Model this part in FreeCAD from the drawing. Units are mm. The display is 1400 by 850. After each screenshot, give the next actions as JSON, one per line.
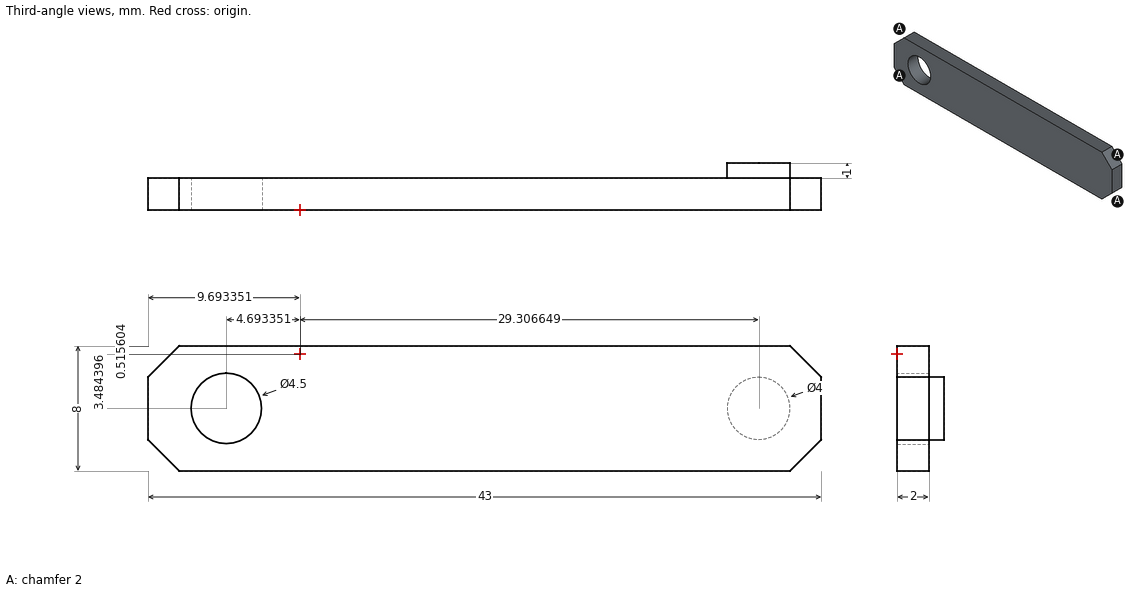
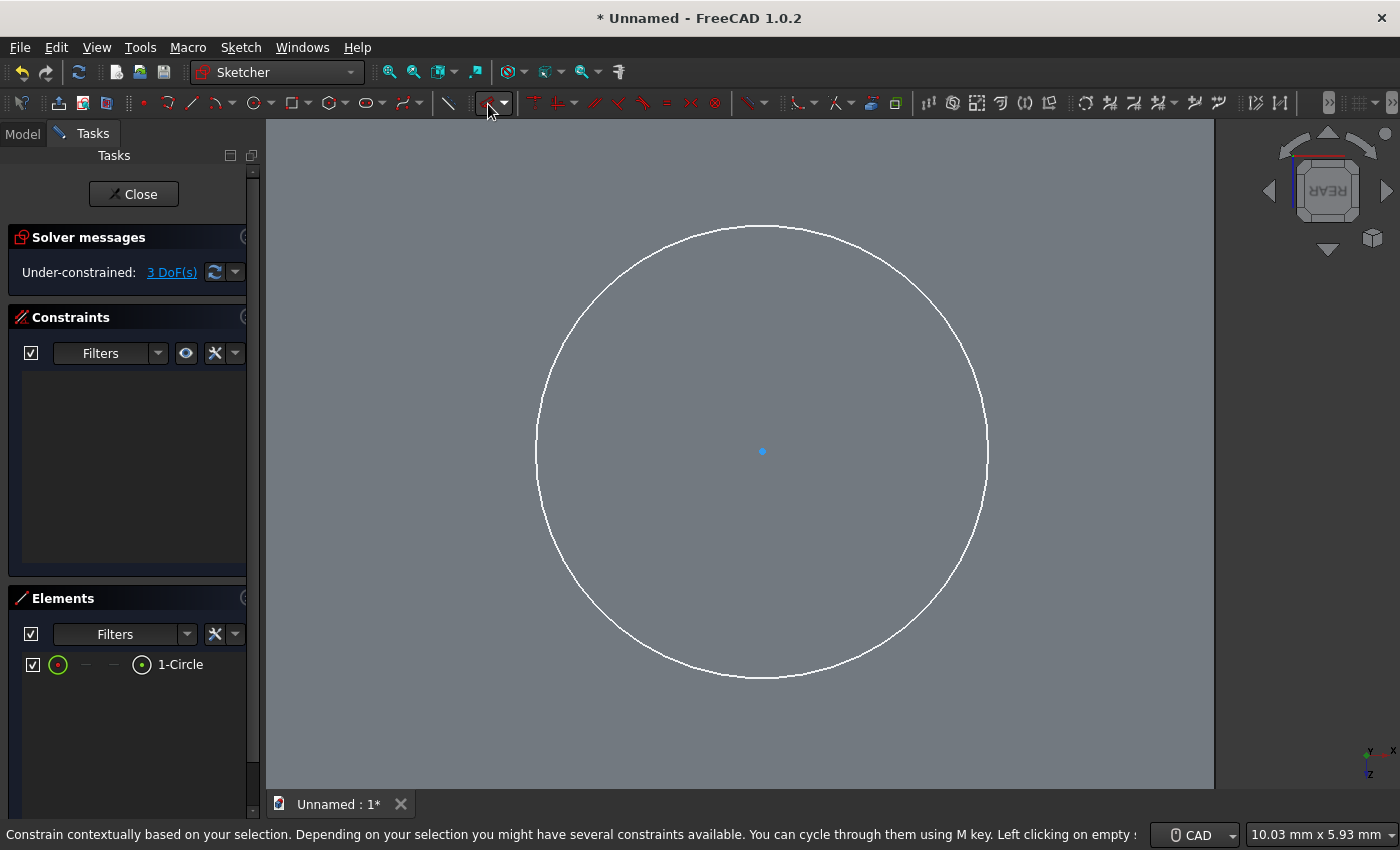
{"action": "left_click", "coordinate": [922, 292]}
{"action": "left_click", "coordinate": [945, 269]}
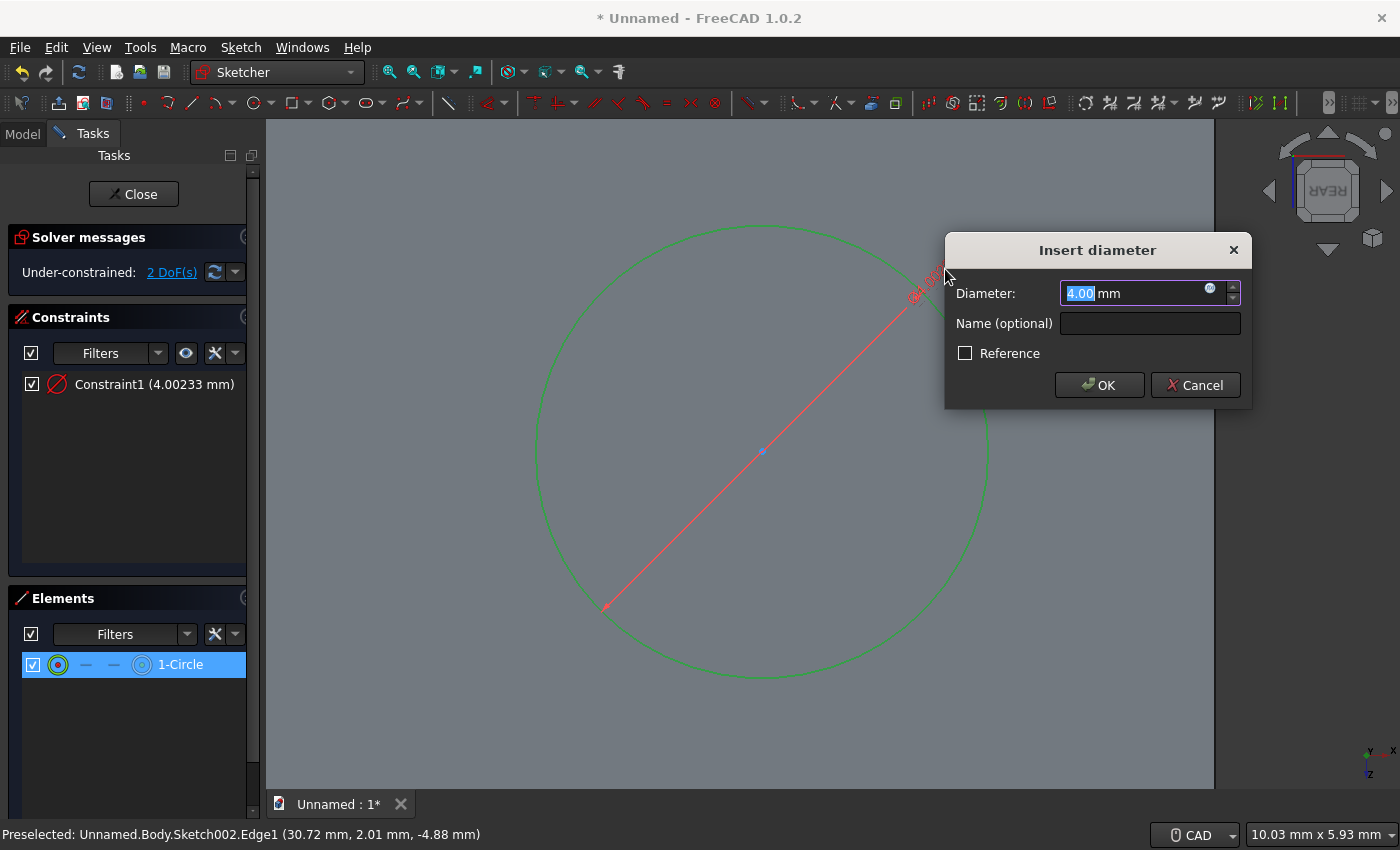
{"action": "type", "text": "4"}
{"action": "key", "text": "Return"}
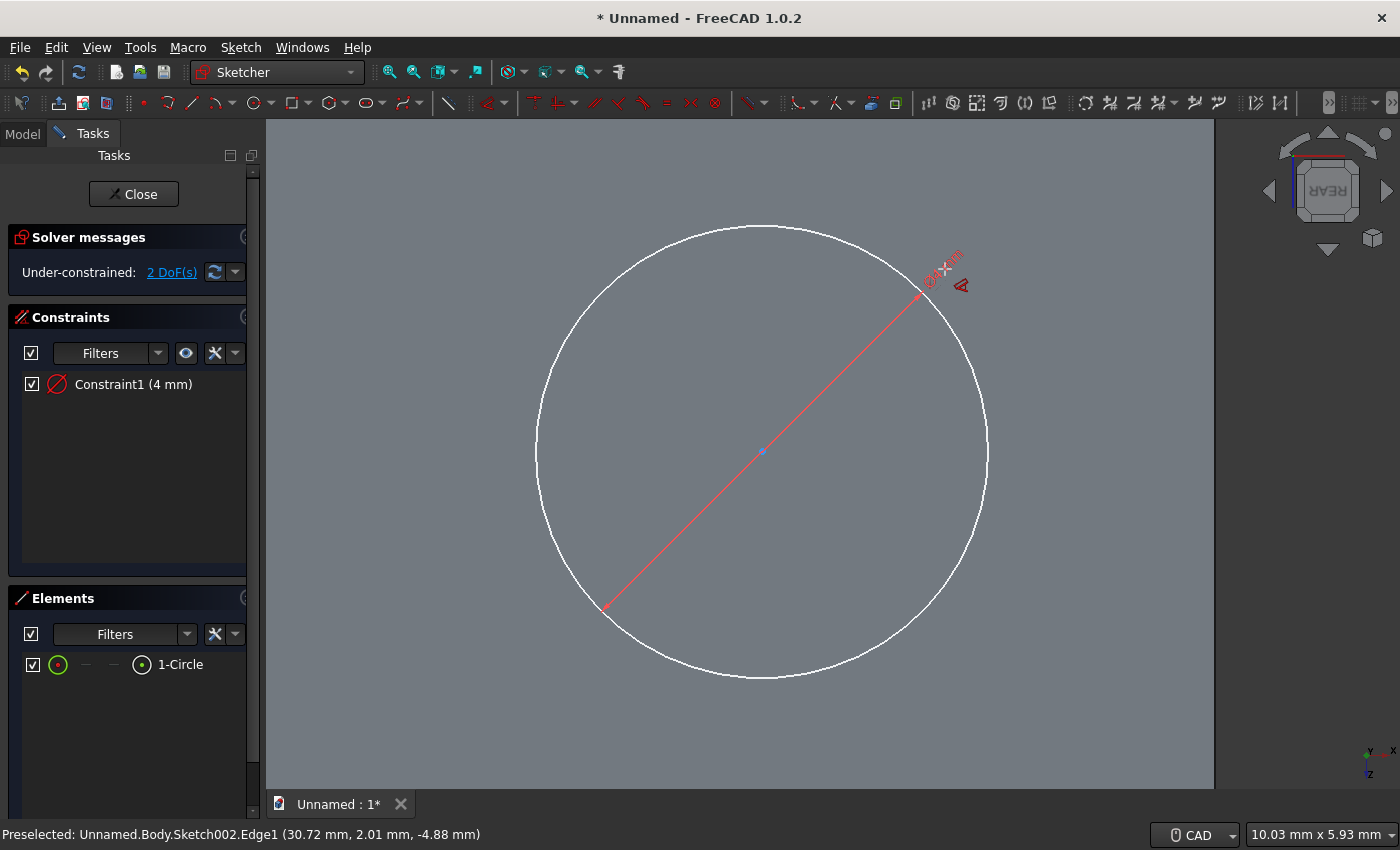
{"action": "left_click", "coordinate": [762, 452]}
{"action": "left_click", "coordinate": [796, 606]}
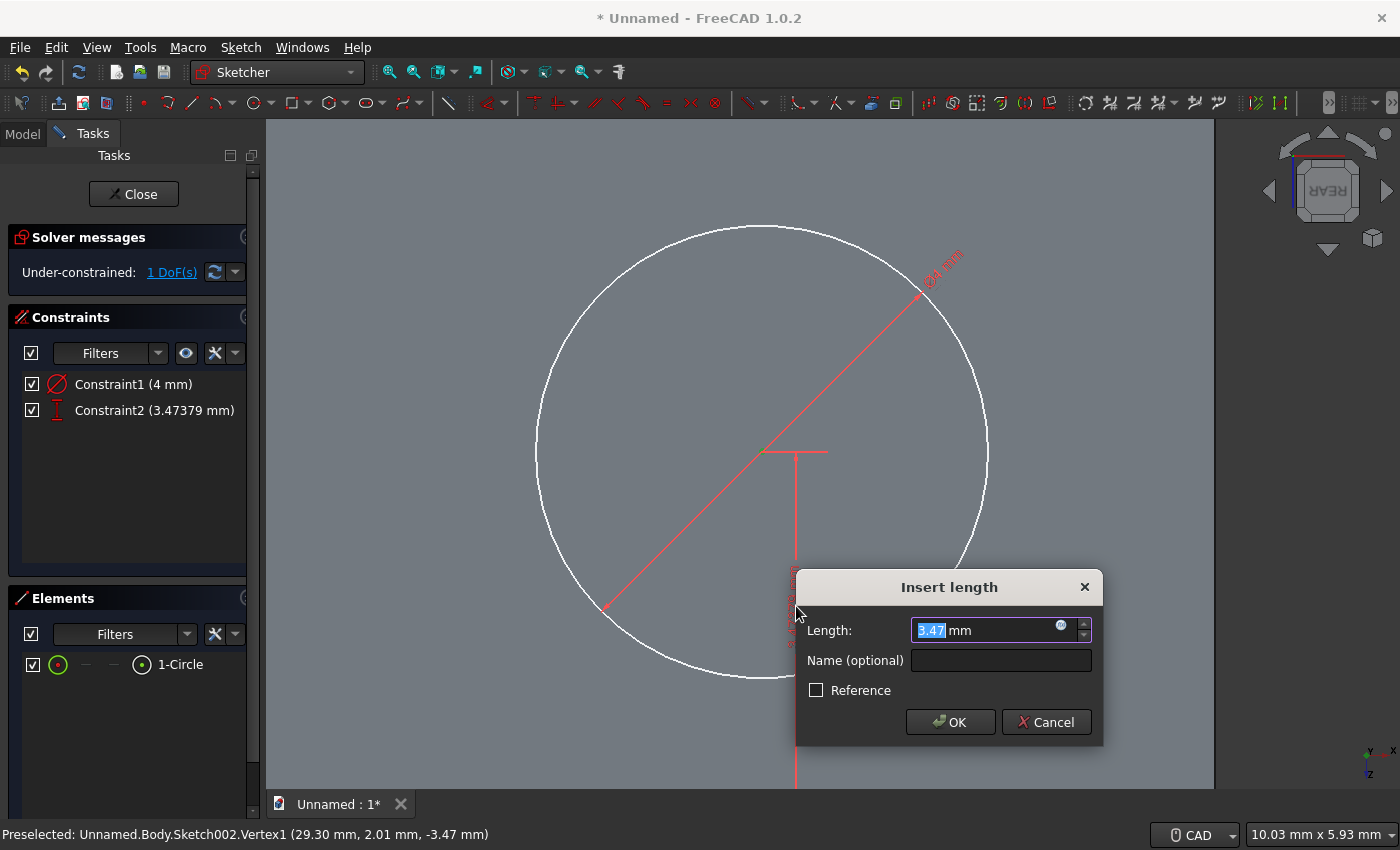
{"action": "type", "text": "3.484396"}
{"action": "key", "text": "Return"}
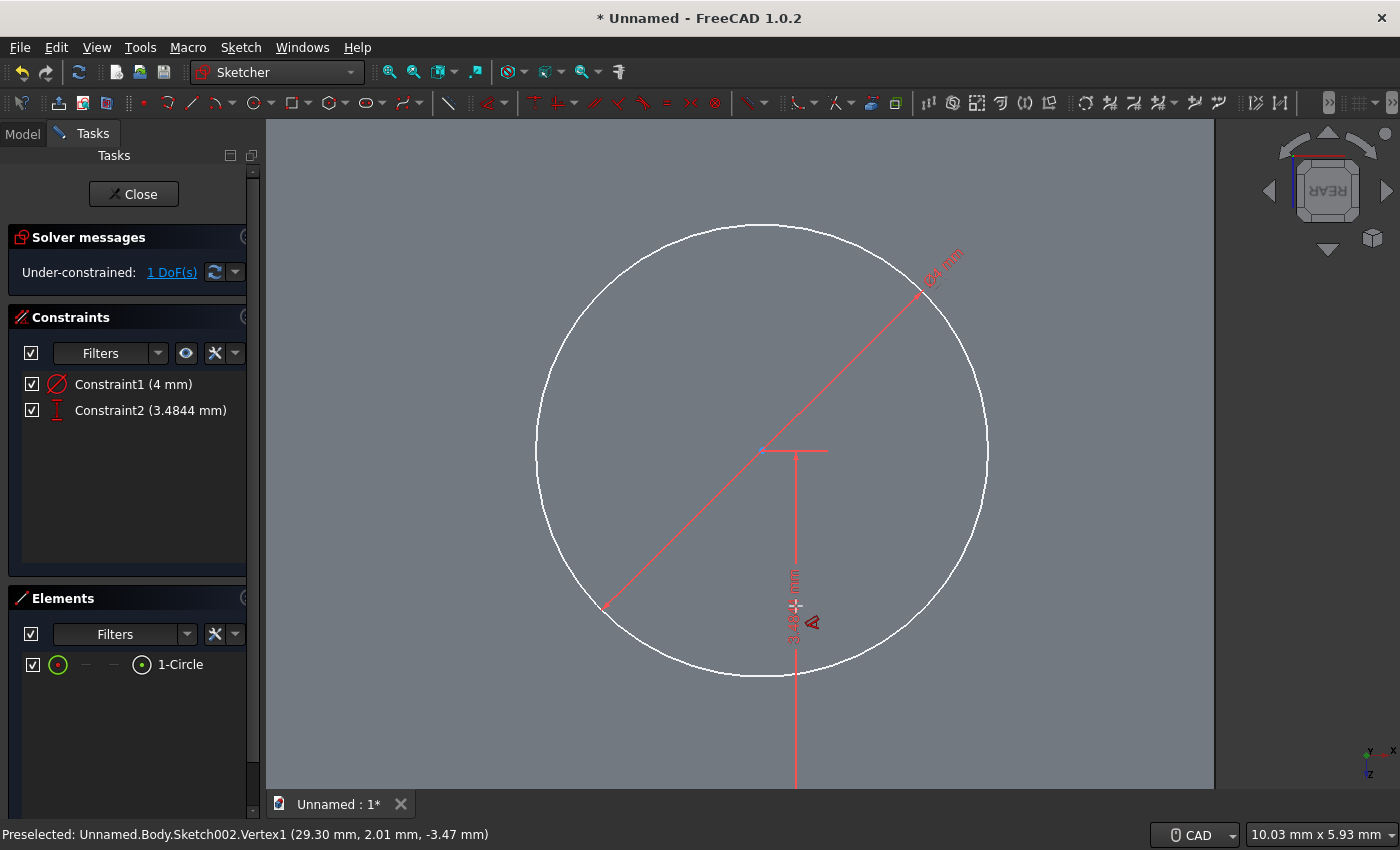
{"action": "left_click", "coordinate": [762, 451]}
{"action": "left_click", "coordinate": [420, 417]}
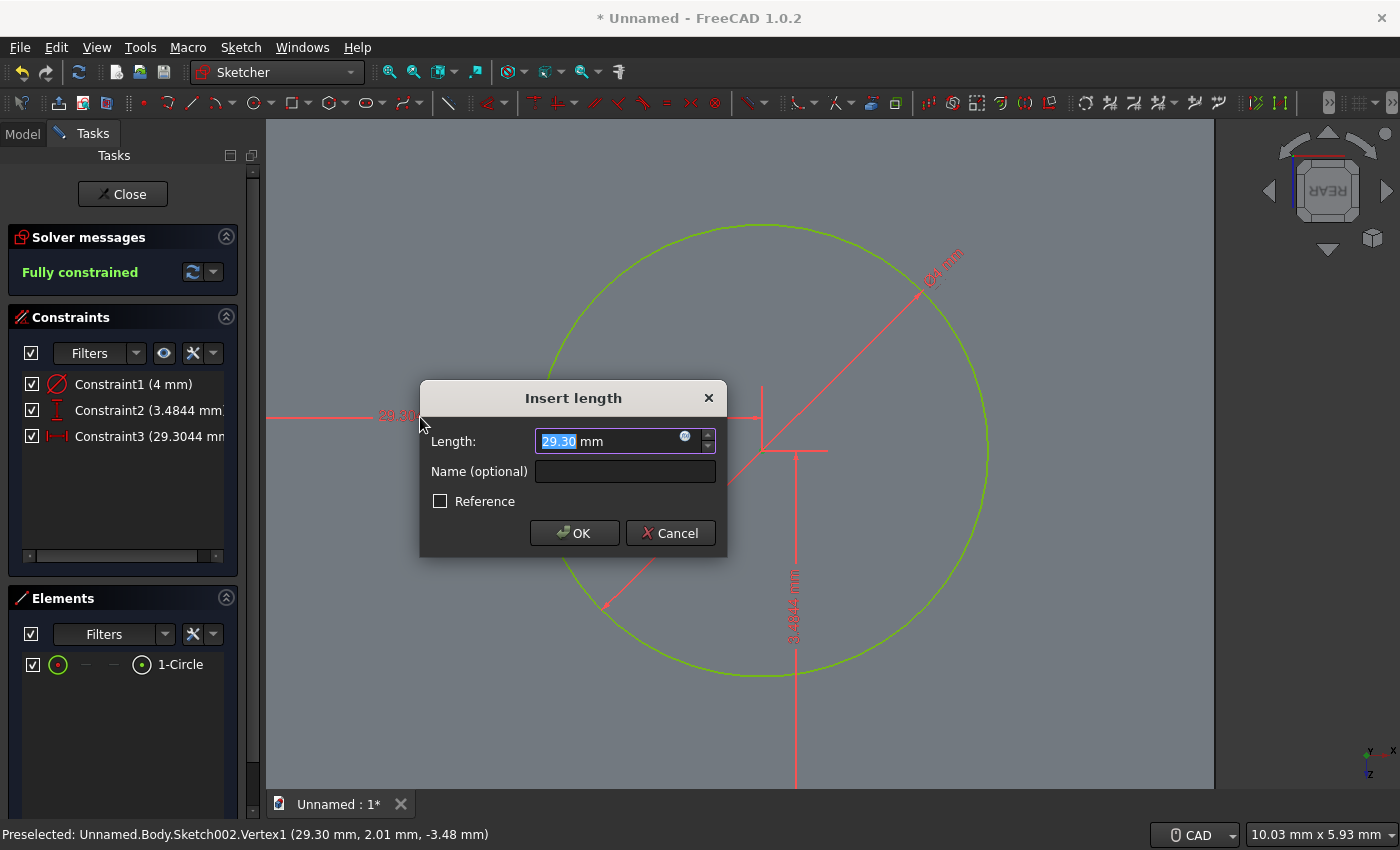
{"action": "type", "text": "29.306649"}
{"action": "key", "text": "Return"}
{"action": "key", "text": "Escape"}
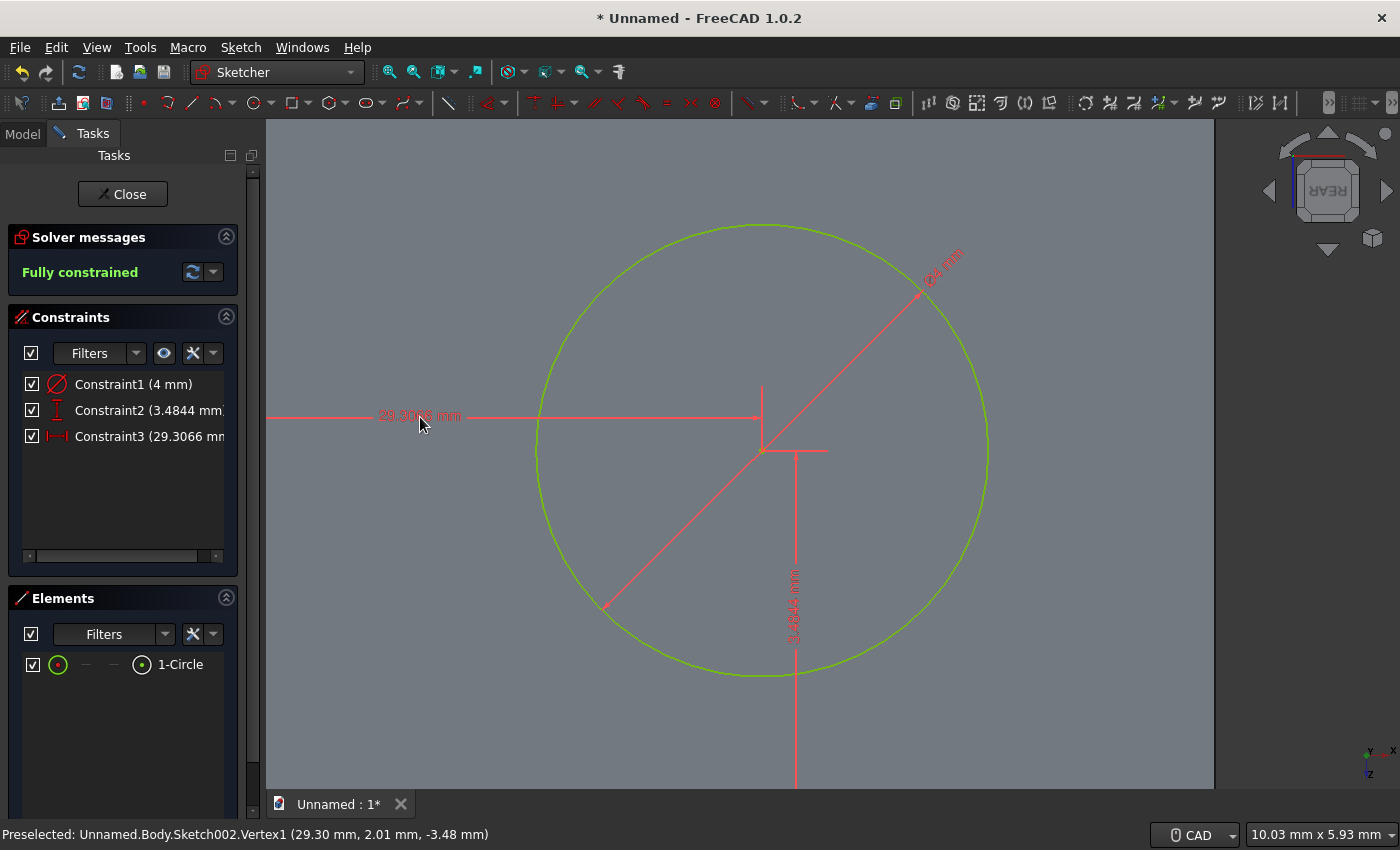
{"action": "left_click", "coordinate": [123, 194]}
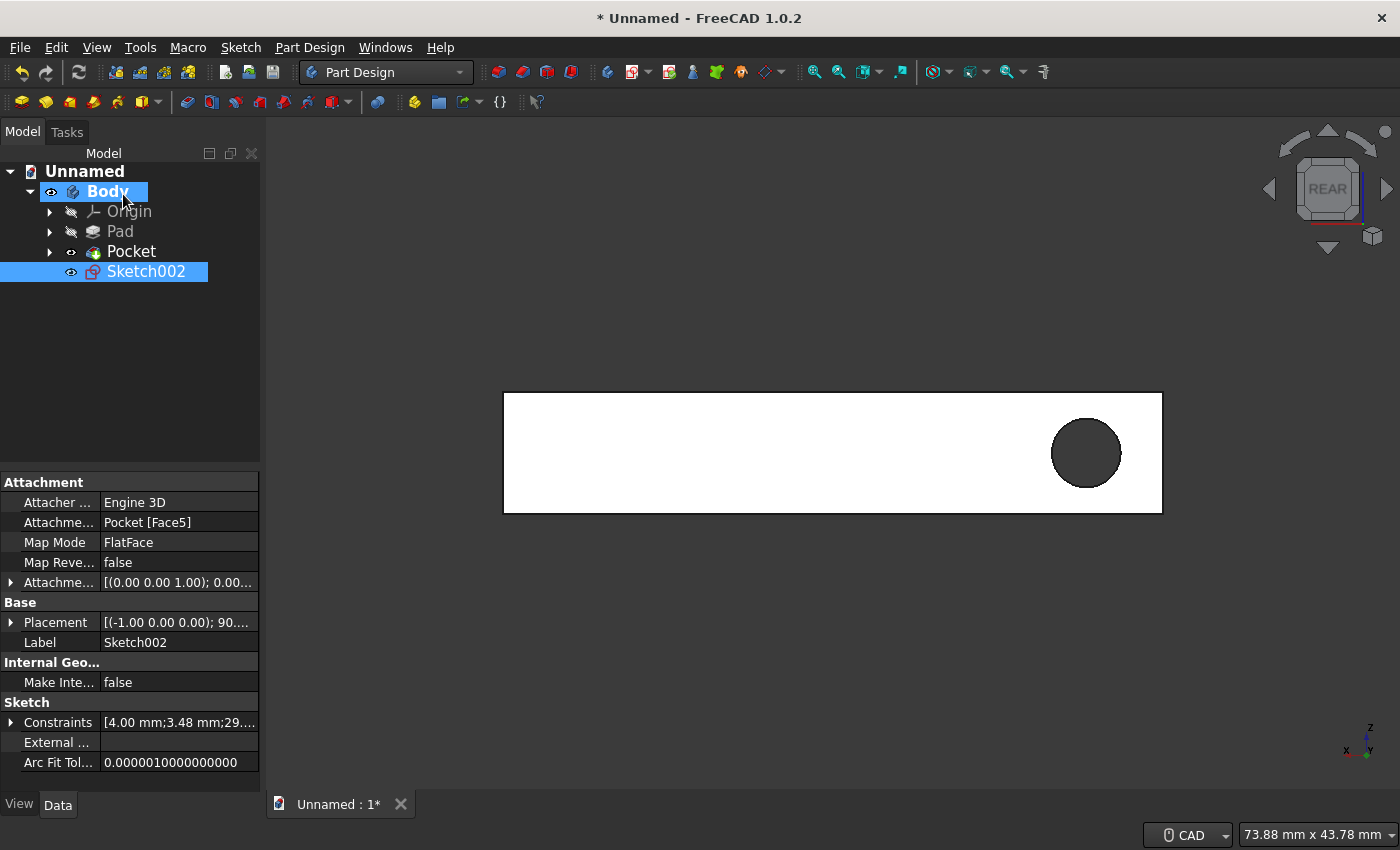
{"action": "left_click", "coordinate": [22, 102]}